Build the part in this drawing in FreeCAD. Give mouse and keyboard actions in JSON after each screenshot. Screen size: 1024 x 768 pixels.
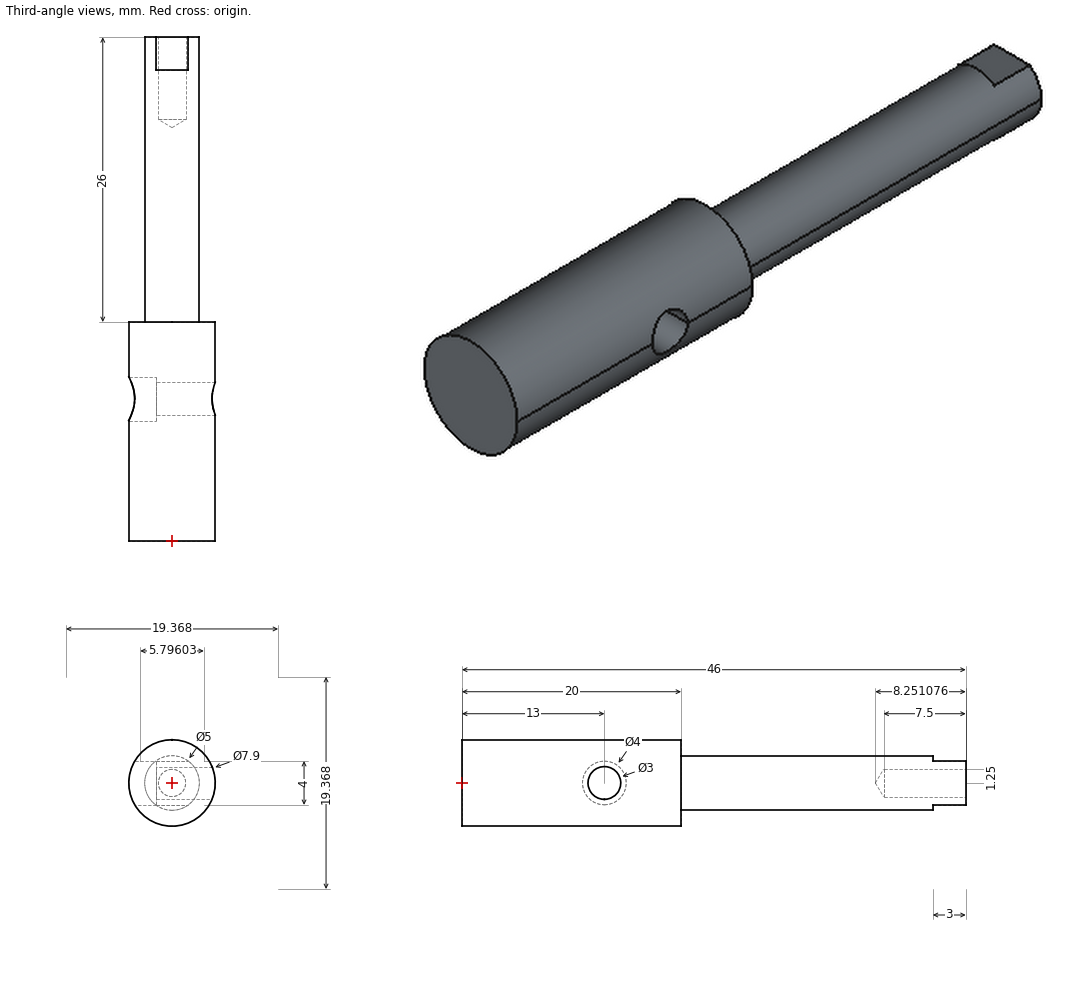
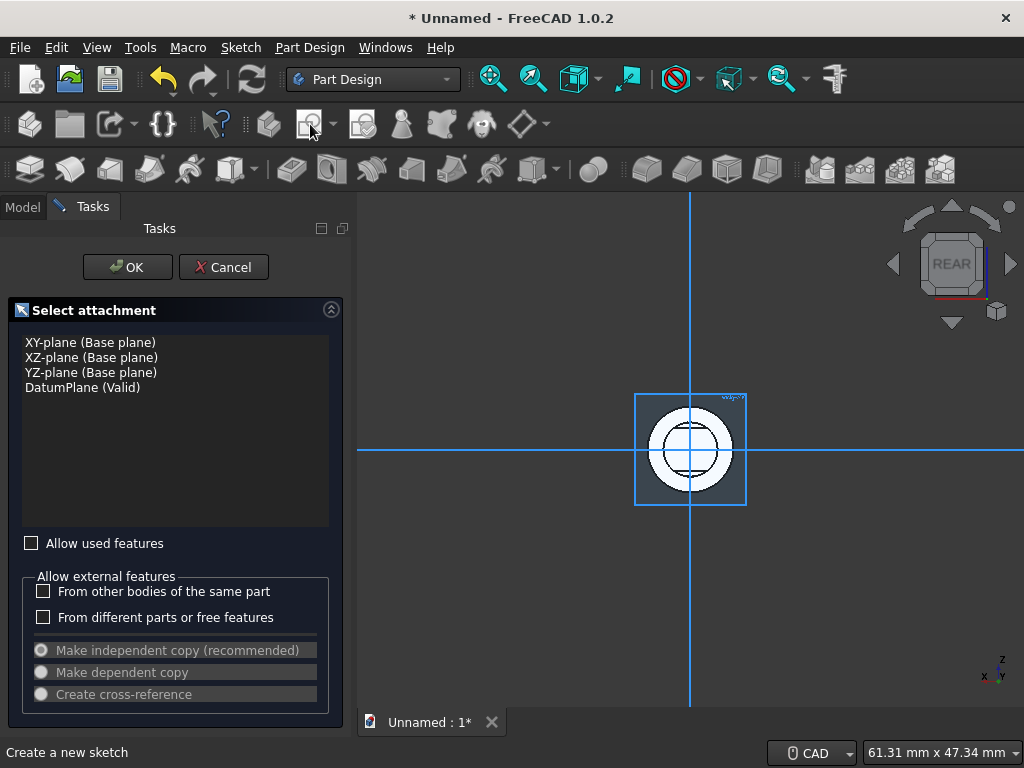
{"action": "left_click", "coordinate": [82, 372]}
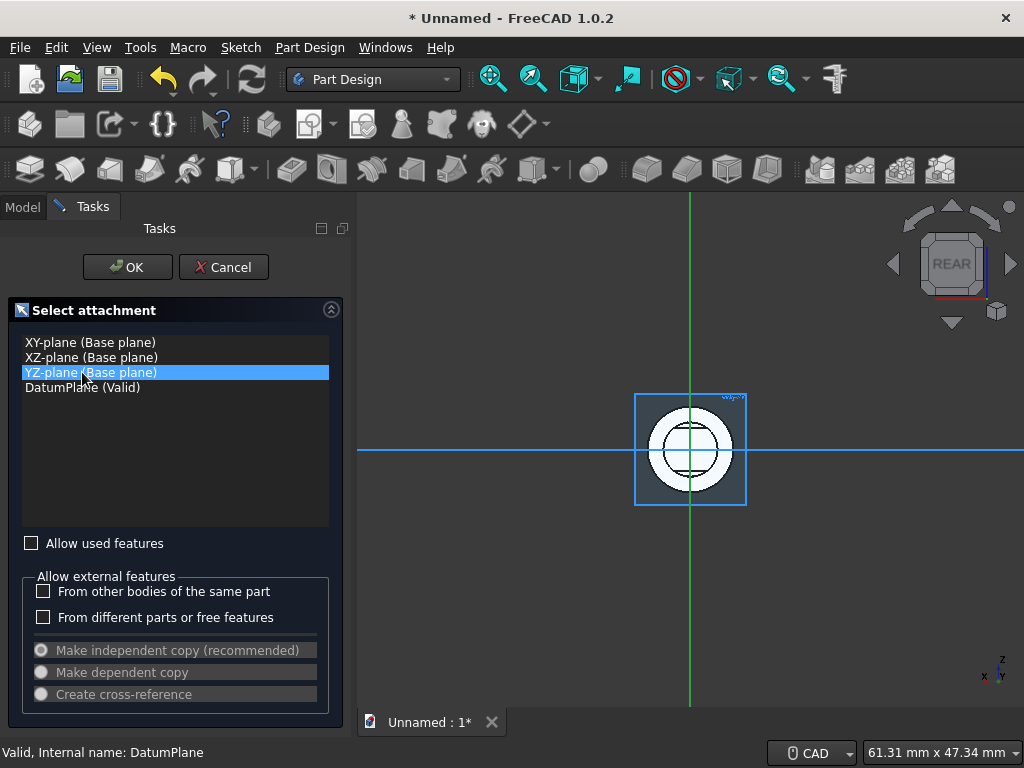
{"action": "left_click", "coordinate": [128, 267]}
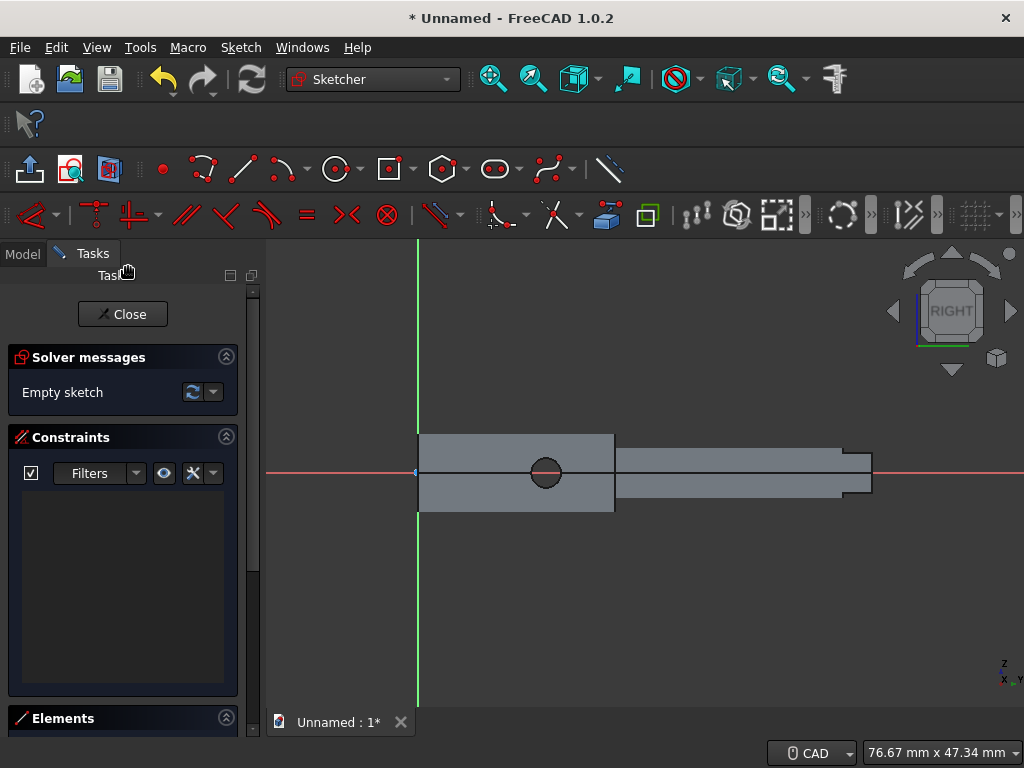
{"action": "left_click", "coordinate": [110, 170]}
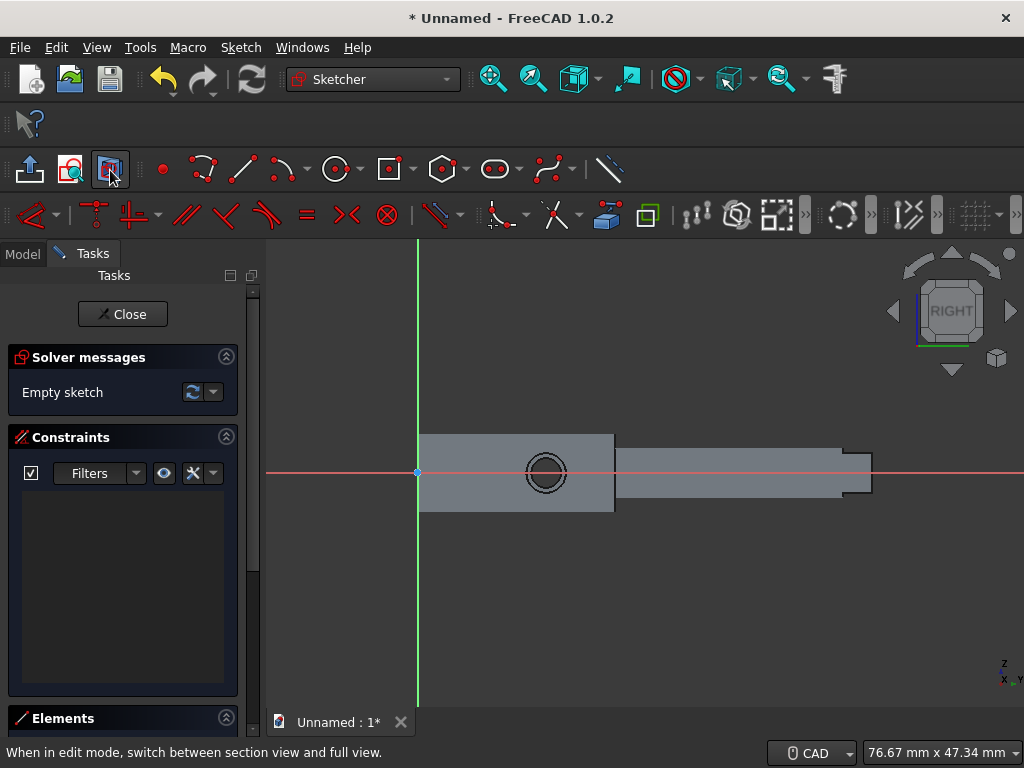
{"action": "scroll", "coordinate": [576, 473], "scroll_direction": "down", "scroll_amount": 5}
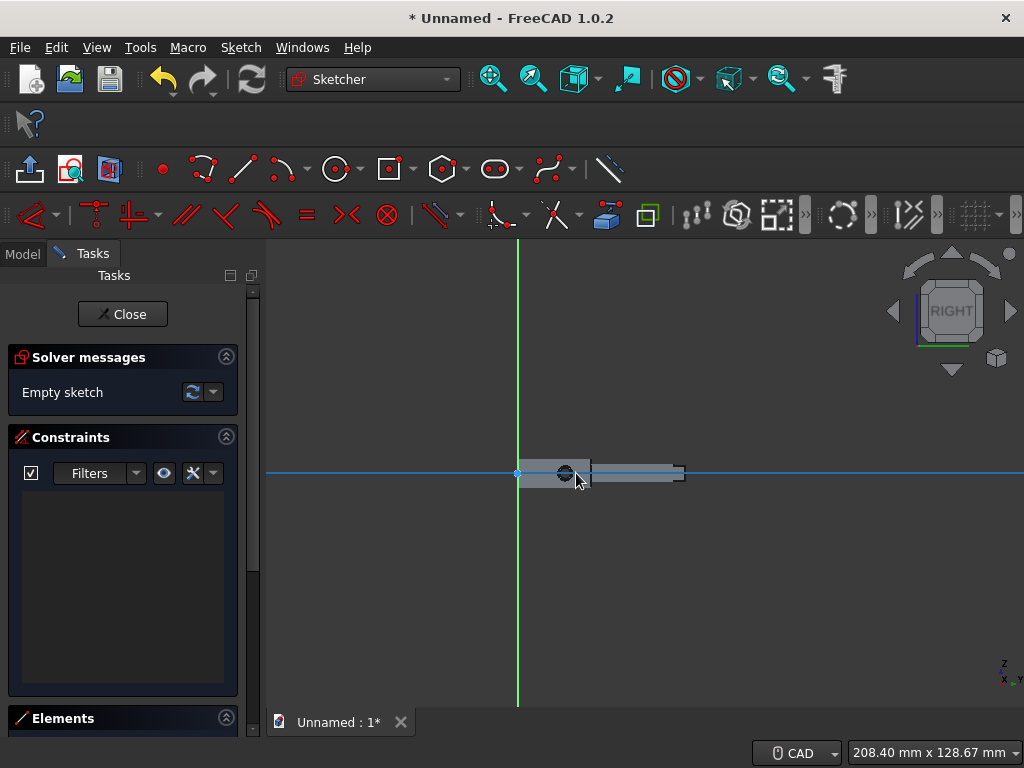
{"action": "scroll", "coordinate": [678, 471], "scroll_direction": "up", "scroll_amount": 13}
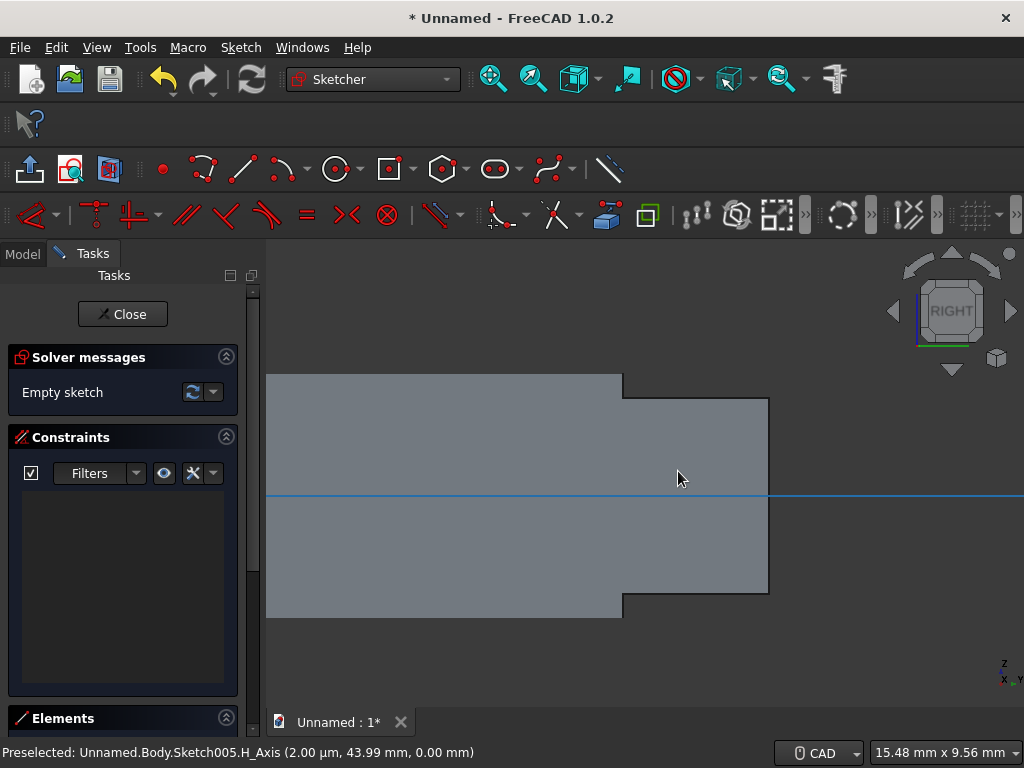
{"action": "left_click", "coordinate": [204, 170]}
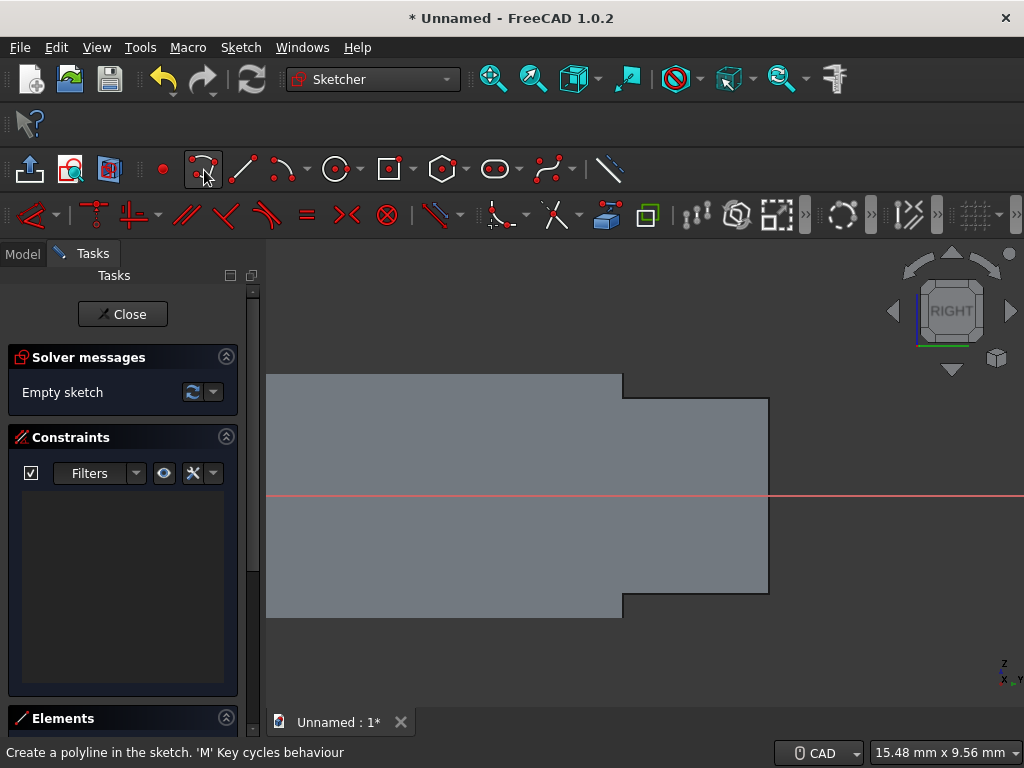
{"action": "left_click", "coordinate": [365, 496]}
{"action": "left_click", "coordinate": [769, 487]}
{"action": "left_click", "coordinate": [769, 435]}
{"action": "left_click", "coordinate": [402, 435]}
{"action": "left_click", "coordinate": [365, 496]}
{"action": "key", "text": "Escape"}
{"action": "key", "text": "Escape"}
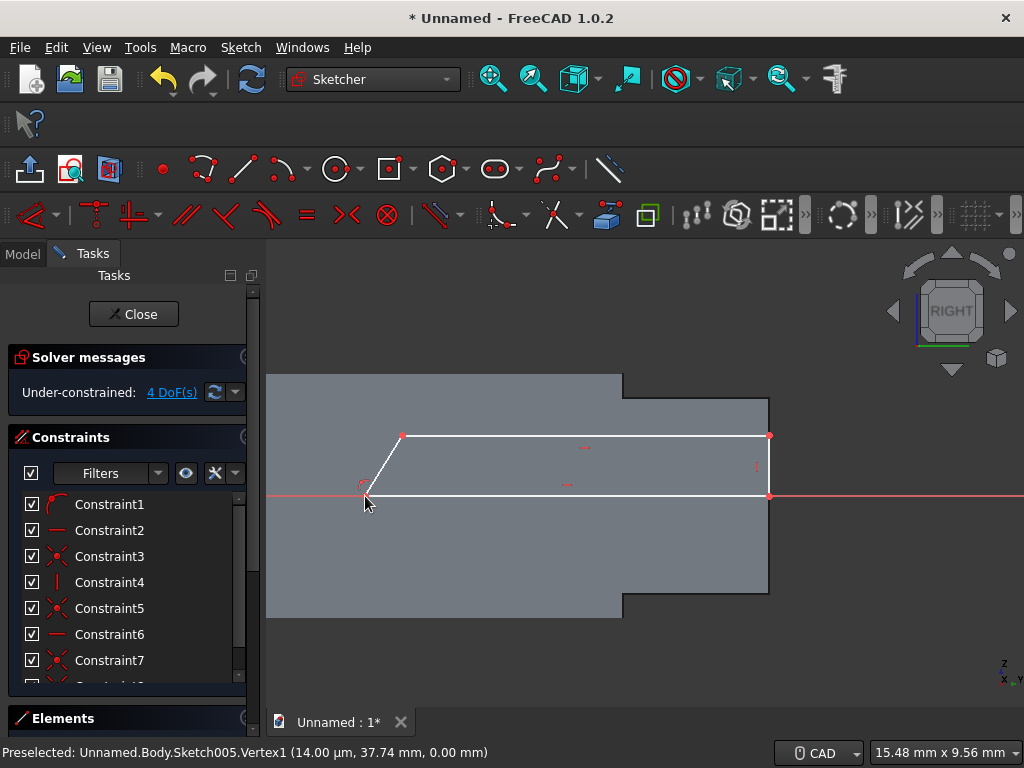
{"action": "left_click", "coordinate": [32, 216]}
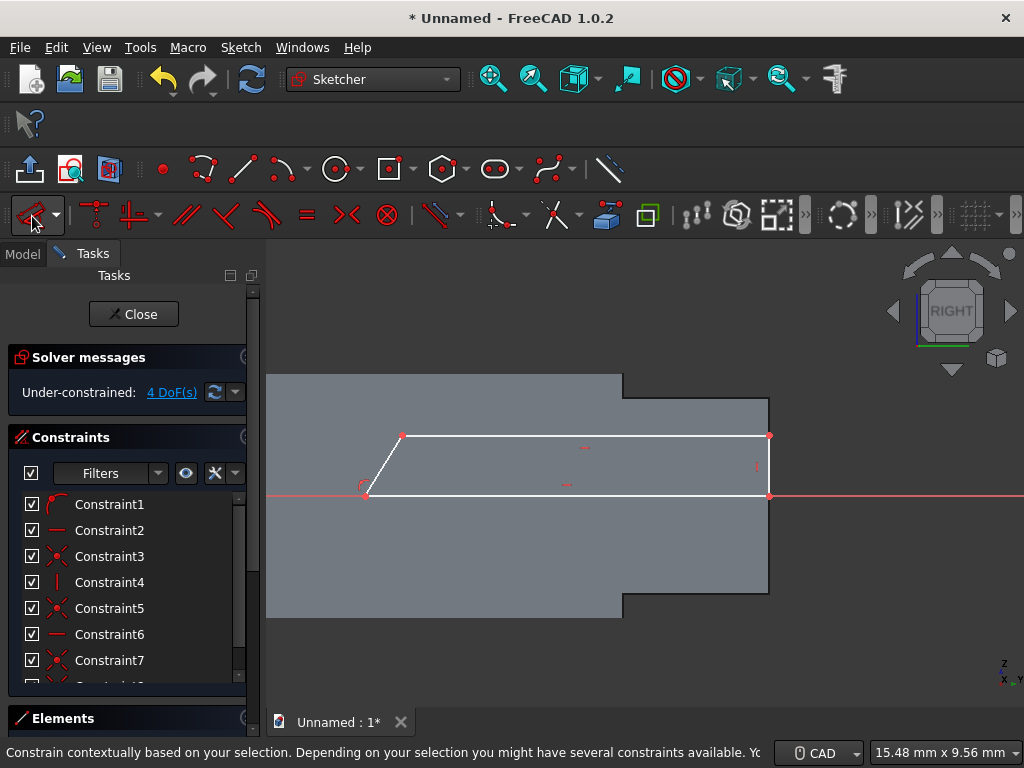
{"action": "left_click", "coordinate": [659, 436]}
{"action": "left_click", "coordinate": [586, 402]}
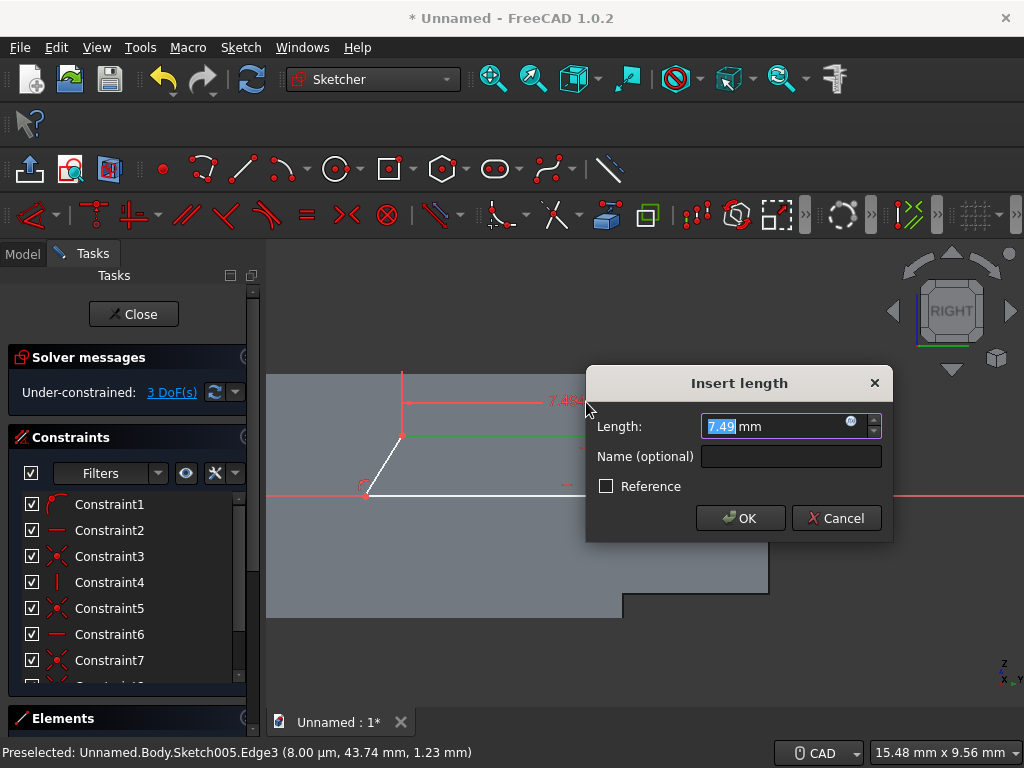
{"action": "type", "text": "7.5"}
{"action": "key", "text": "Return"}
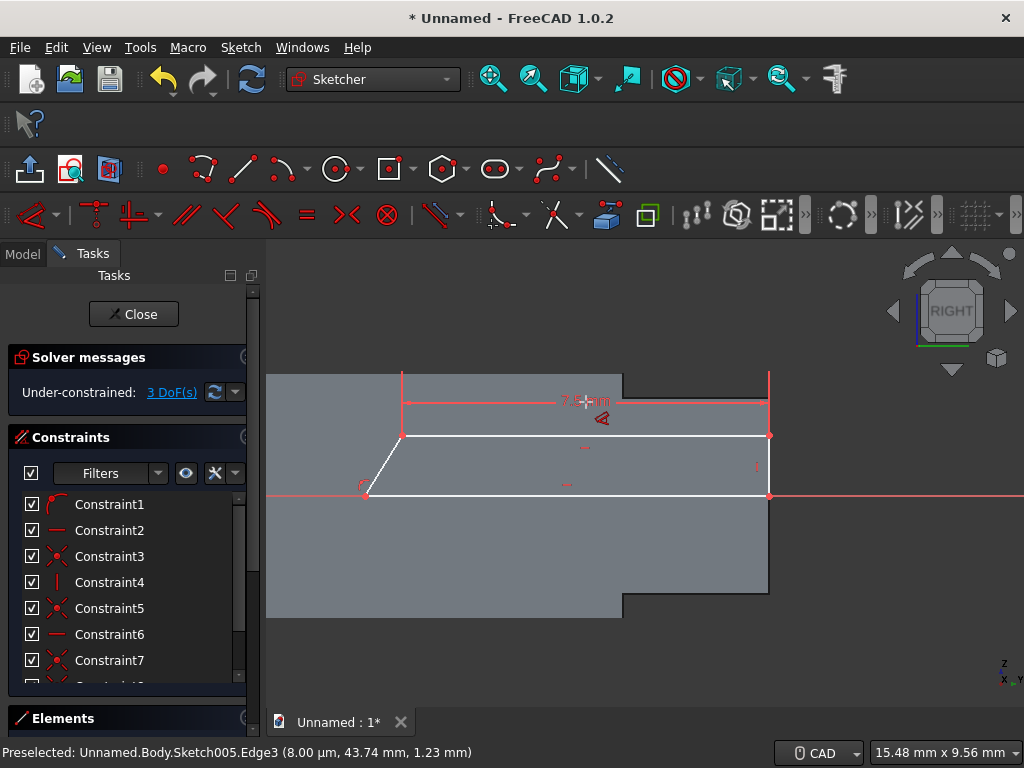
{"action": "left_click", "coordinate": [769, 496]}
{"action": "left_click", "coordinate": [532, 530]}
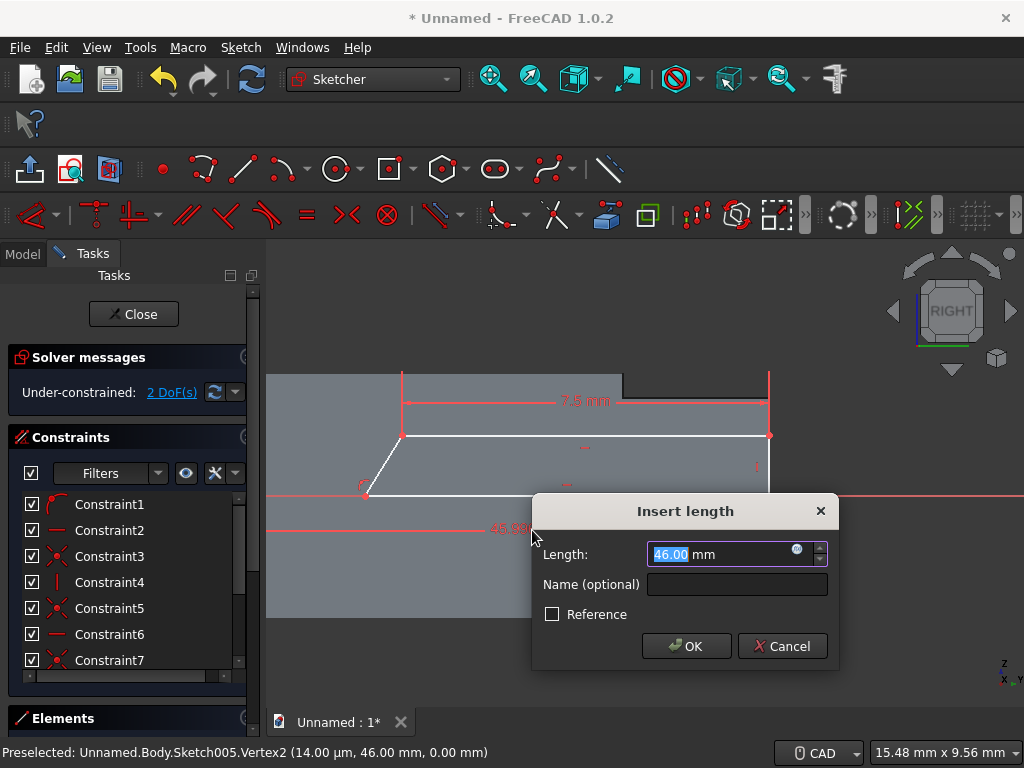
{"action": "type", "text": "46"}
{"action": "key", "text": "Return"}